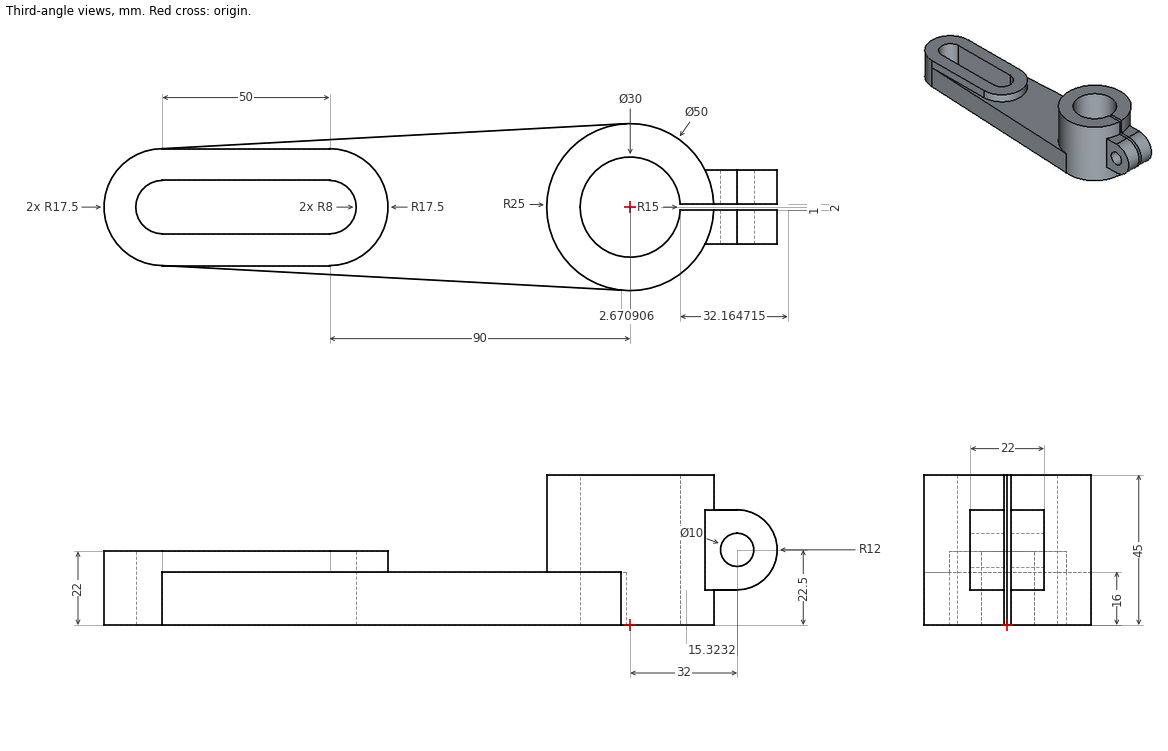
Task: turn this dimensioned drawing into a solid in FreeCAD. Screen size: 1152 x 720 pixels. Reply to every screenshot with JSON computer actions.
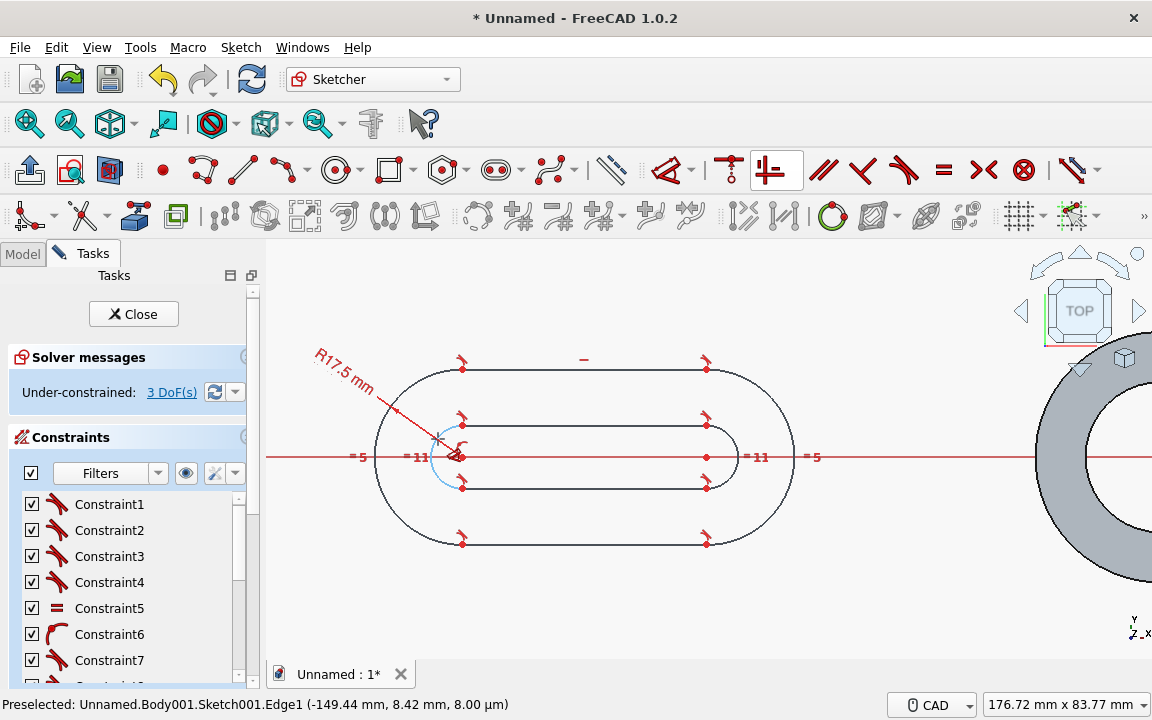
{"action": "left_click", "coordinate": [437, 439]}
{"action": "left_click", "coordinate": [411, 420]}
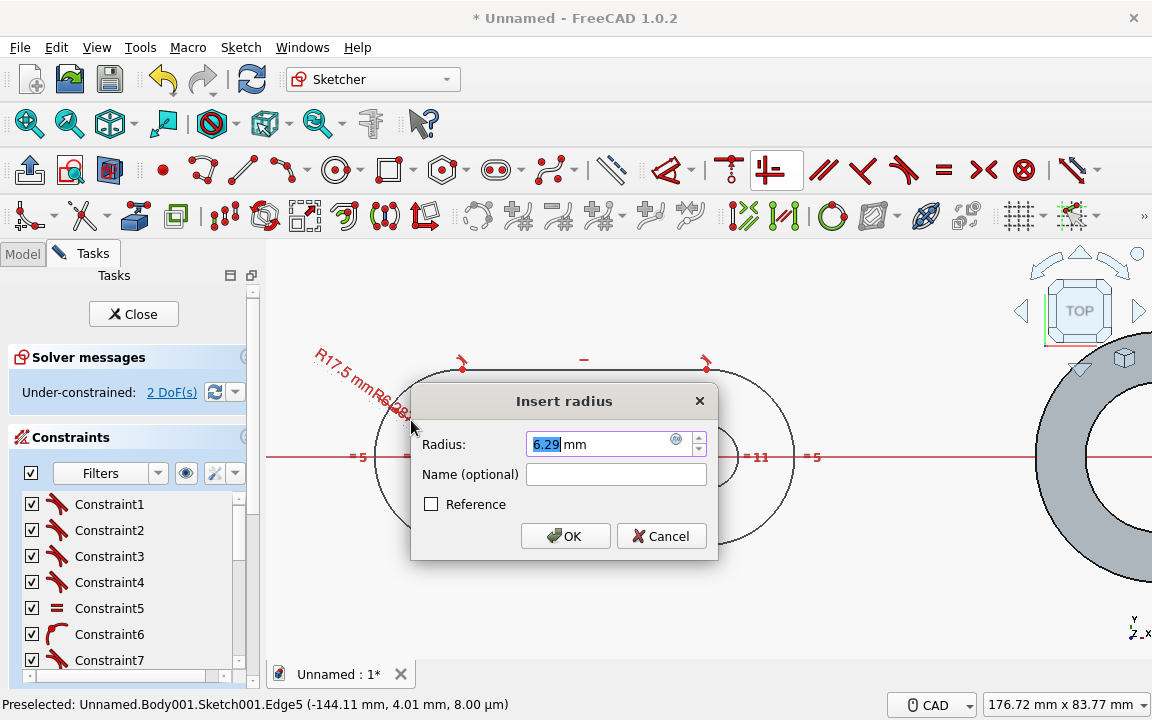
{"action": "type", "text": "8"}
{"action": "key", "text": "Return"}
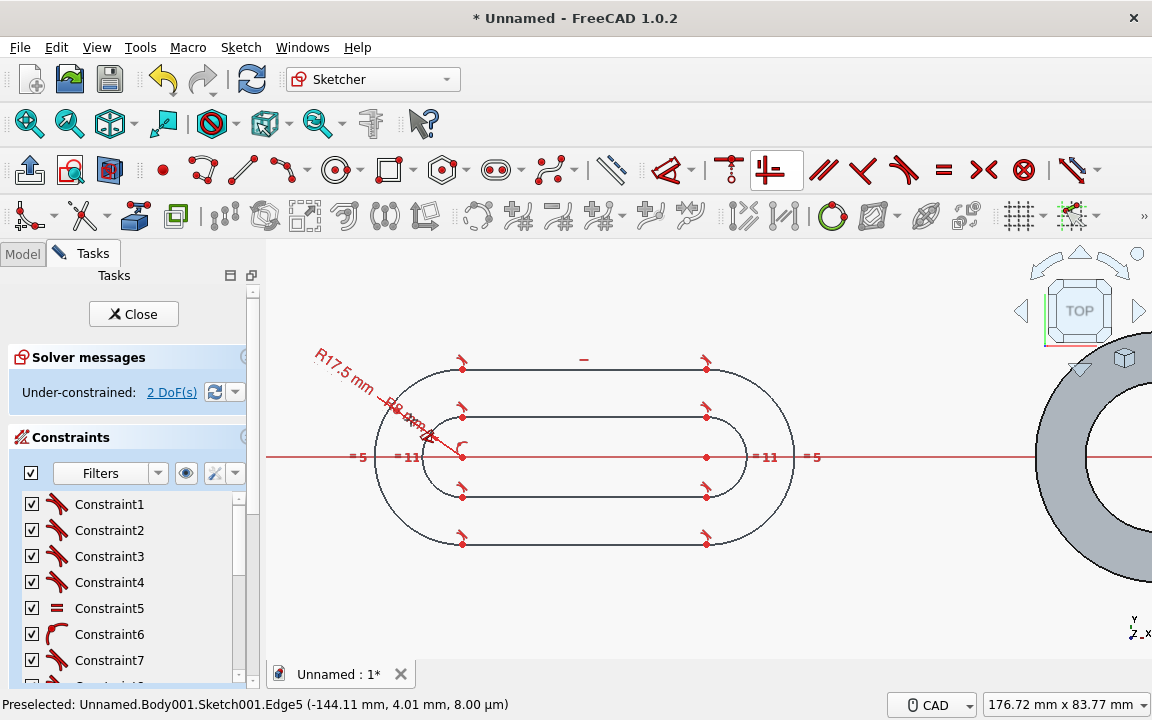
{"action": "left_click", "coordinate": [536, 370]}
{"action": "left_click", "coordinate": [585, 336]}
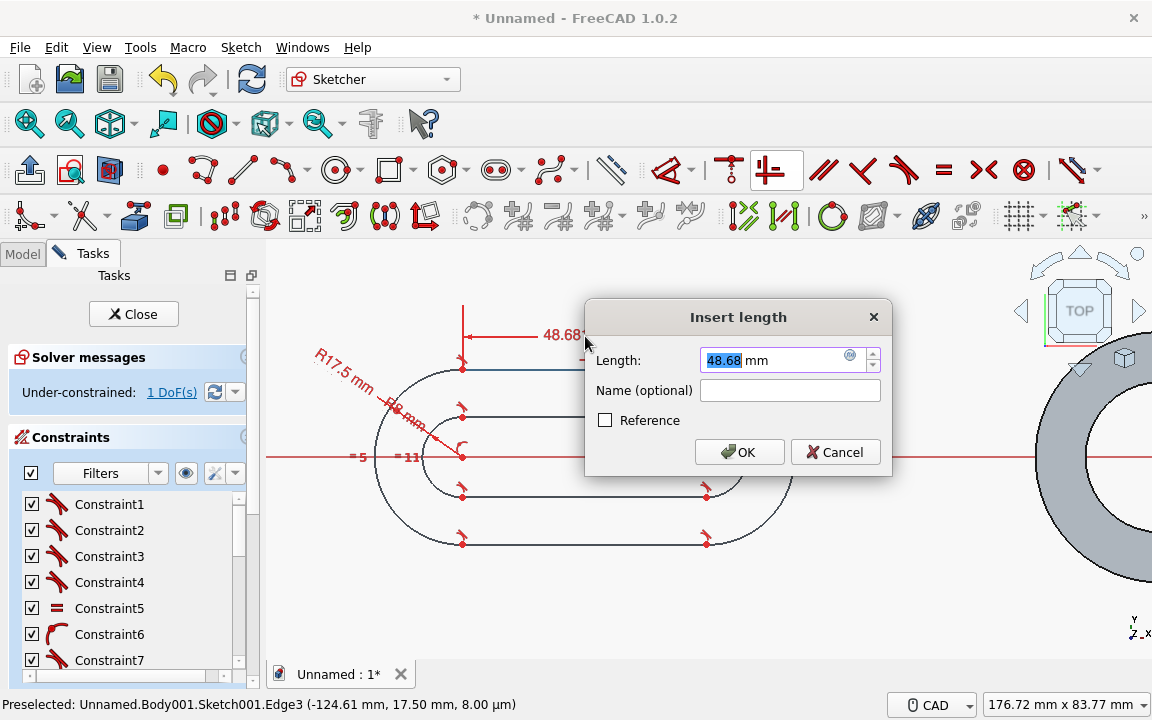
{"action": "type", "text": "50"}
{"action": "key", "text": "Return"}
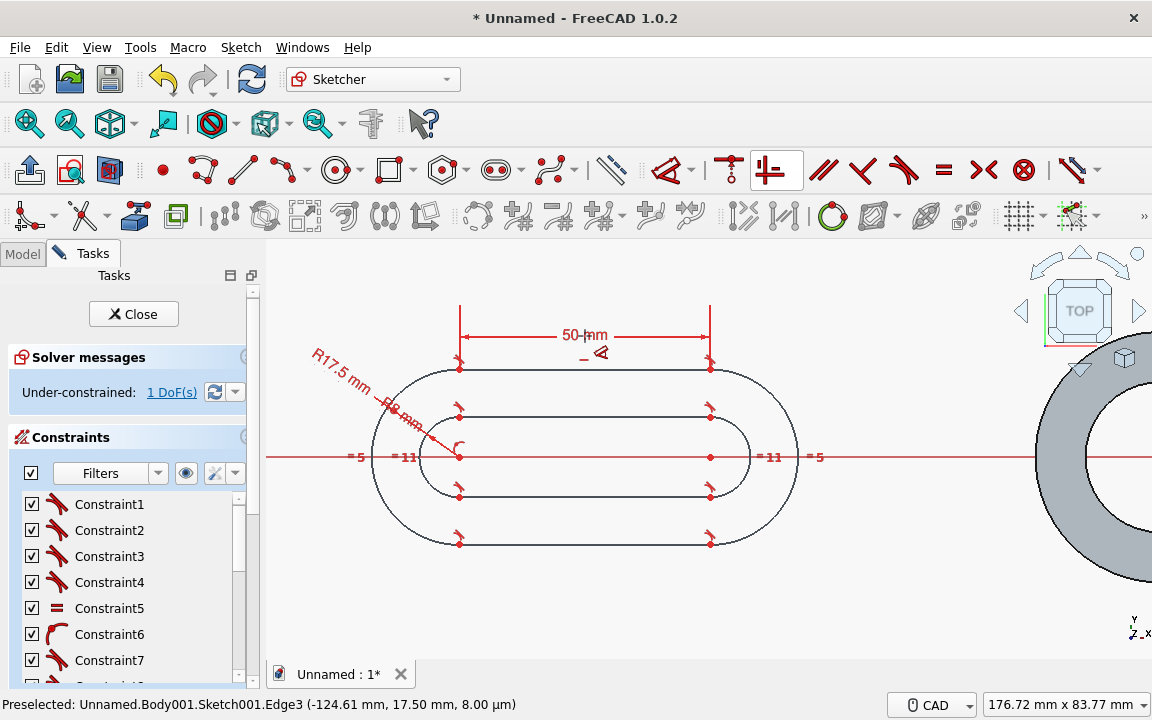
{"action": "left_click", "coordinate": [710, 545]}
{"action": "left_click", "coordinate": [849, 579]}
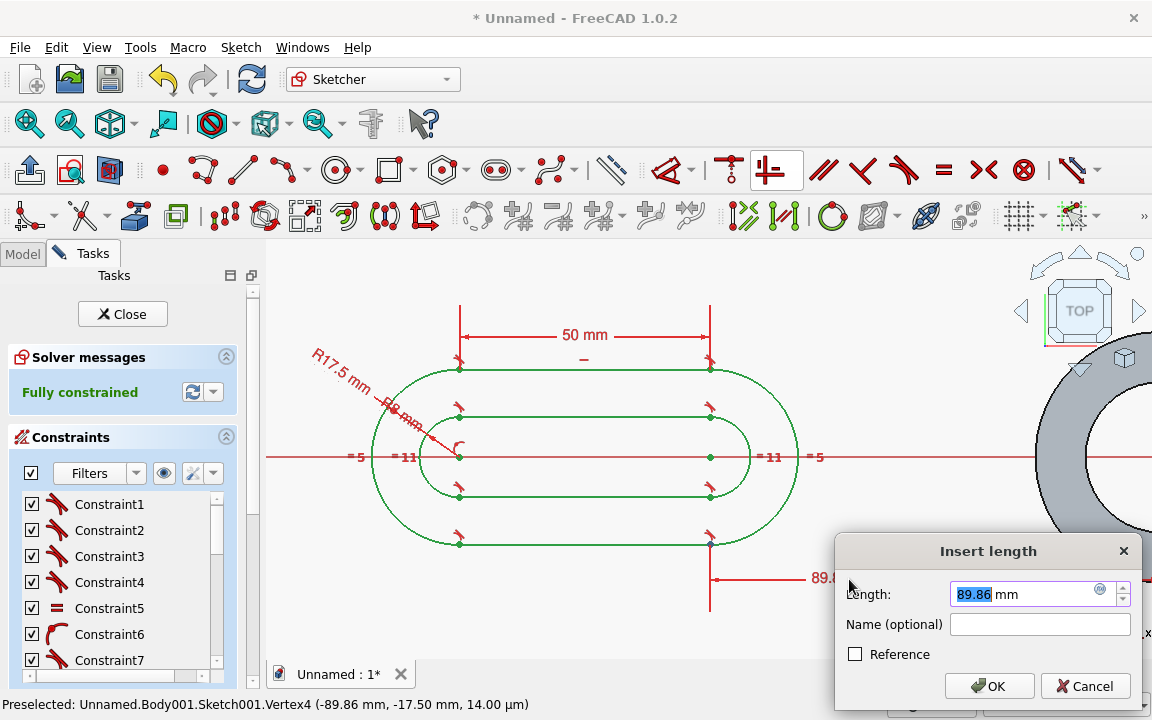
{"action": "type", "text": "90"}
{"action": "key", "text": "Return"}
{"action": "key", "text": "Escape"}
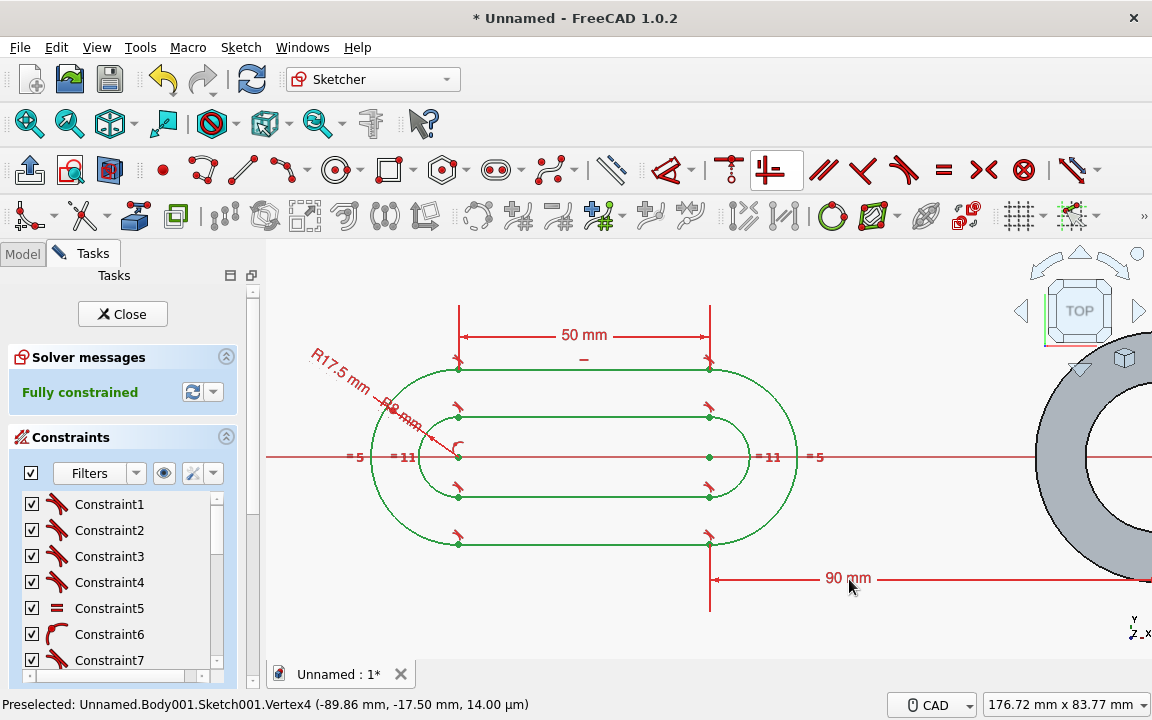
{"action": "left_click", "coordinate": [123, 314]}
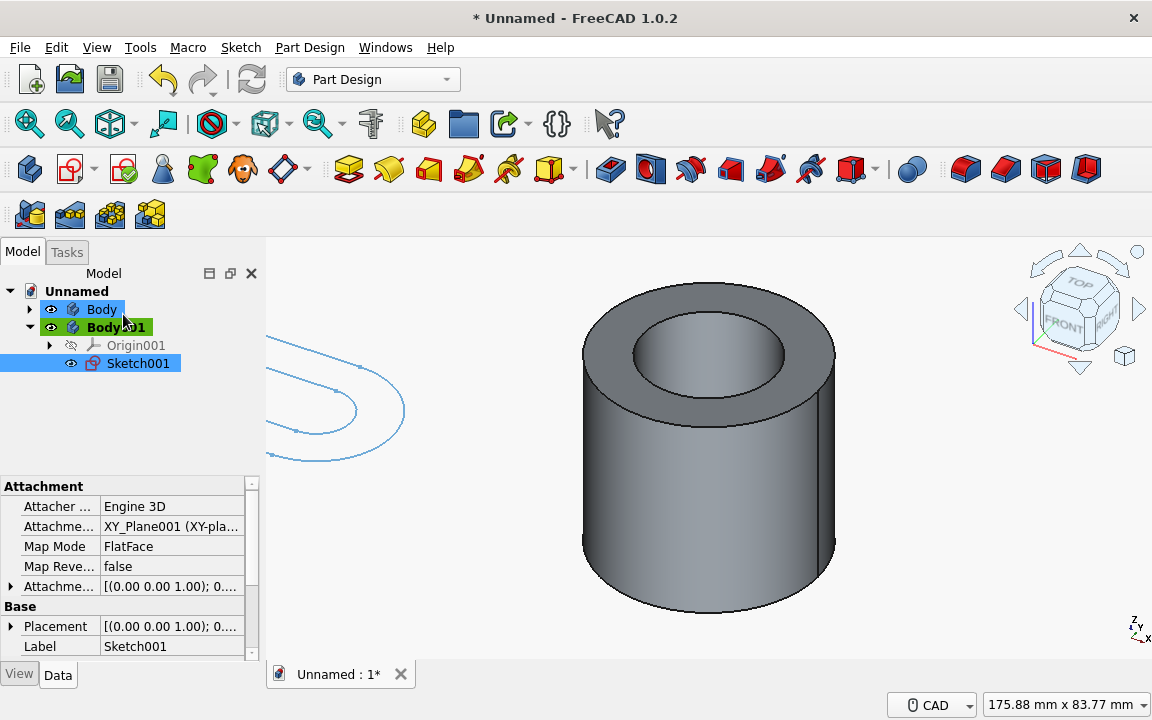
{"action": "left_click", "coordinate": [350, 170]}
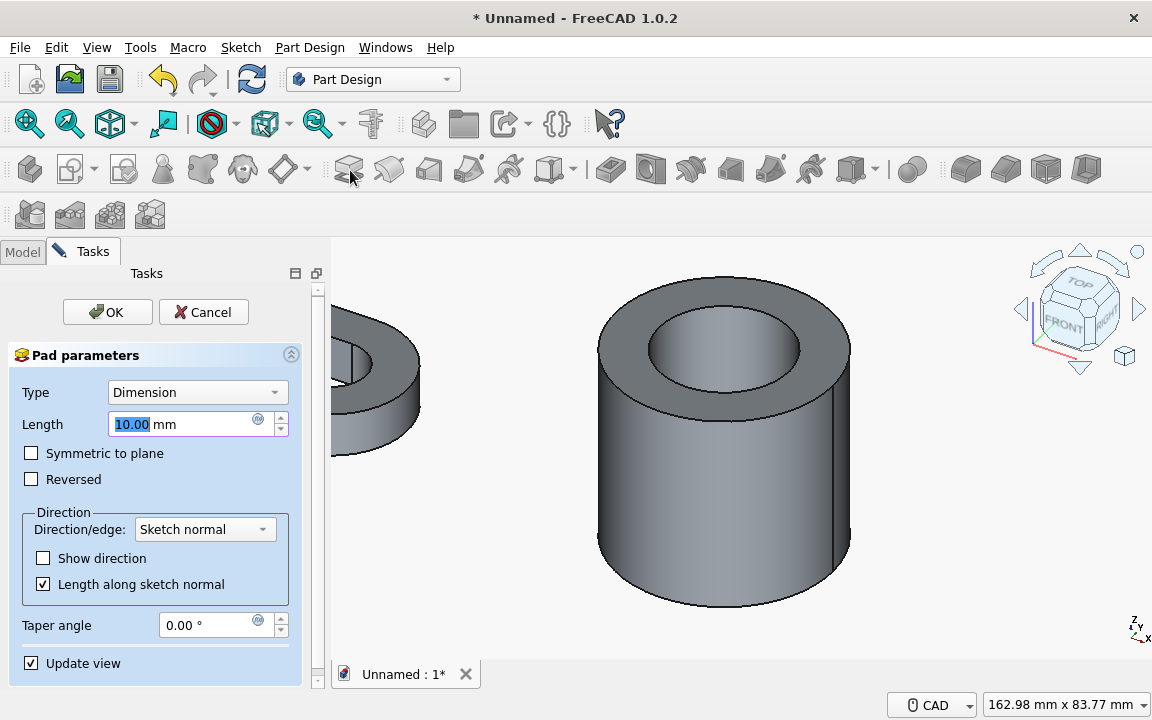
{"action": "type", "text": "22"}
{"action": "key", "text": "Tab"}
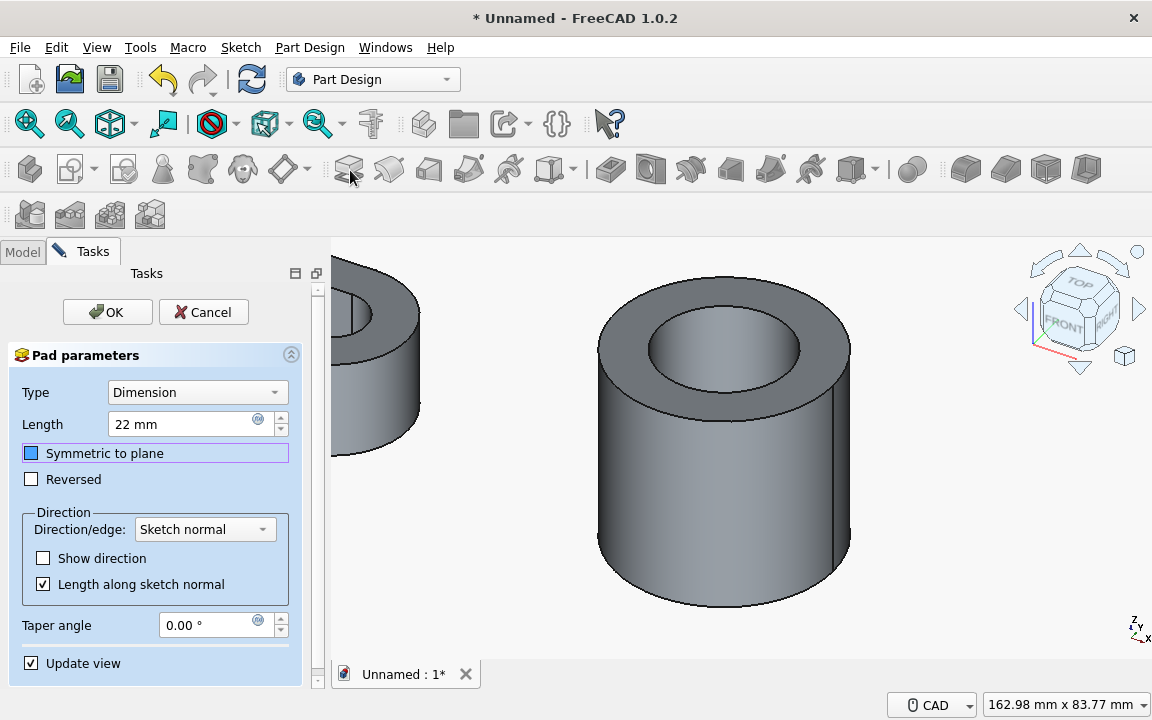
{"action": "left_click", "coordinate": [108, 312]}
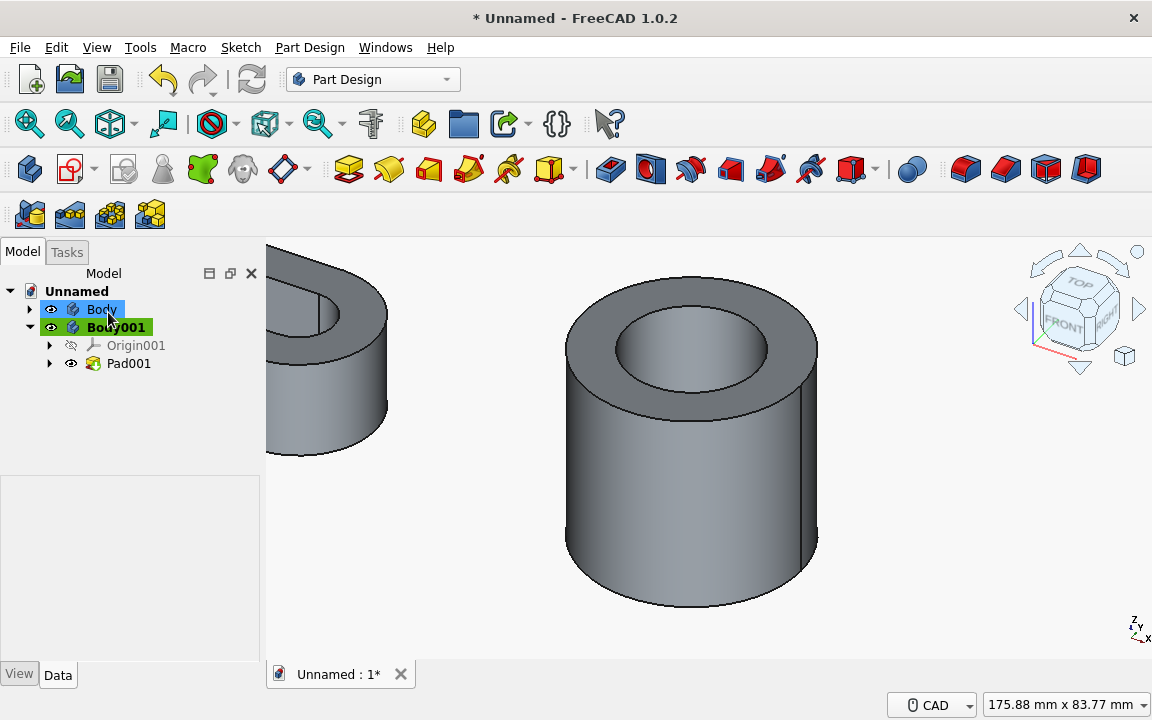
{"action": "left_click", "coordinate": [30, 124]}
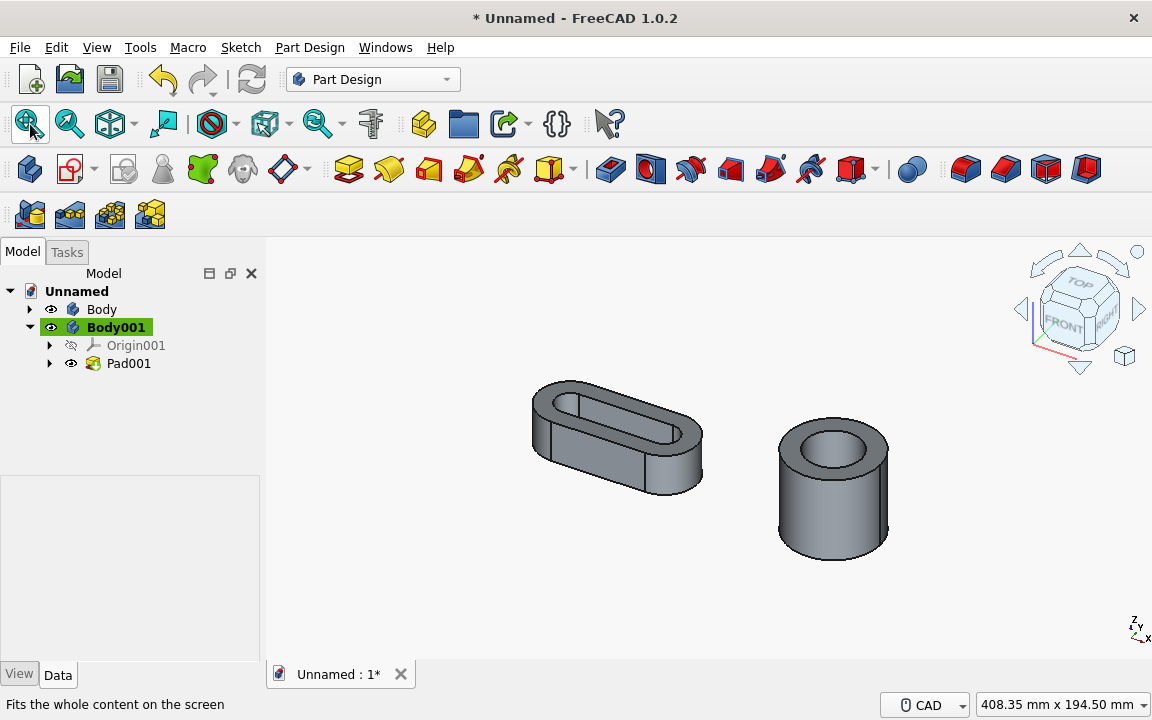
{"action": "double_click", "coordinate": [96, 309]}